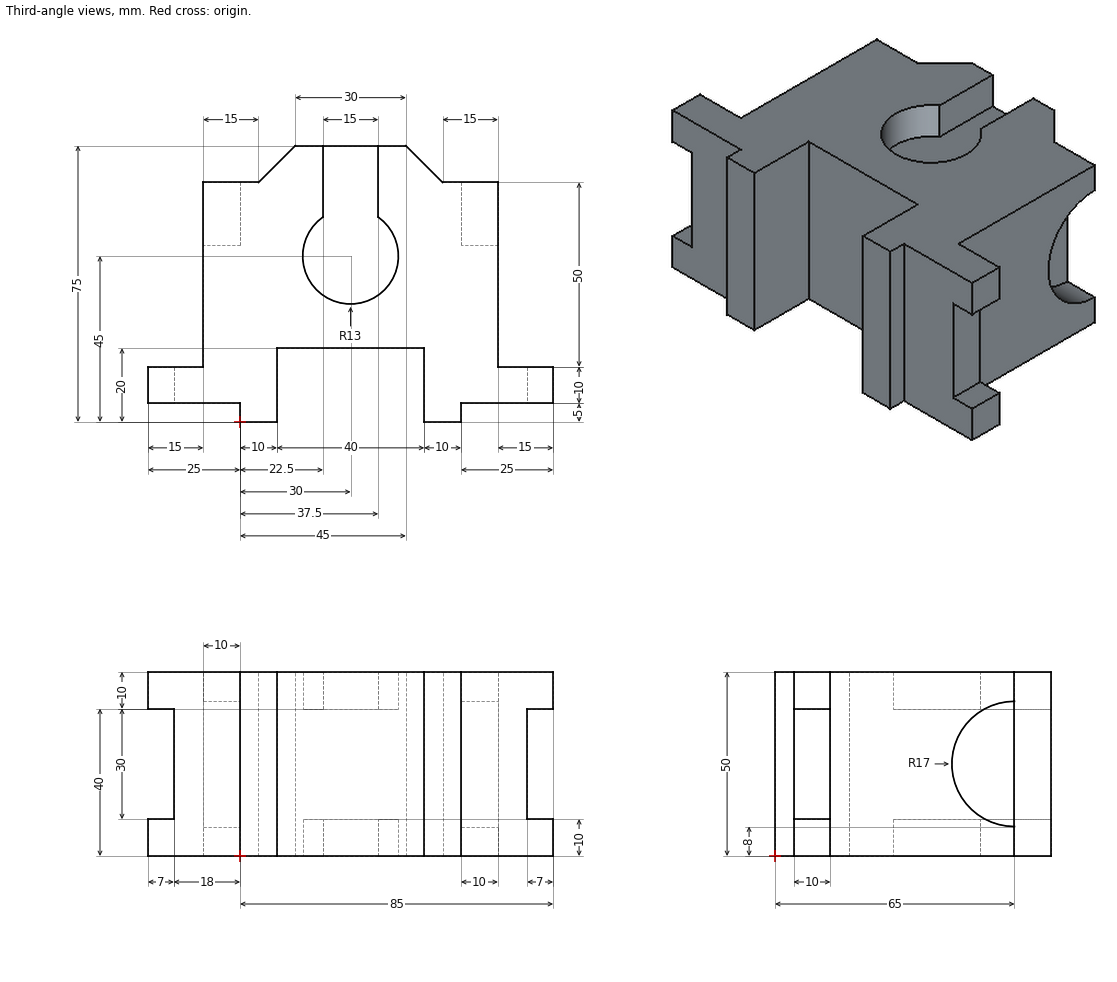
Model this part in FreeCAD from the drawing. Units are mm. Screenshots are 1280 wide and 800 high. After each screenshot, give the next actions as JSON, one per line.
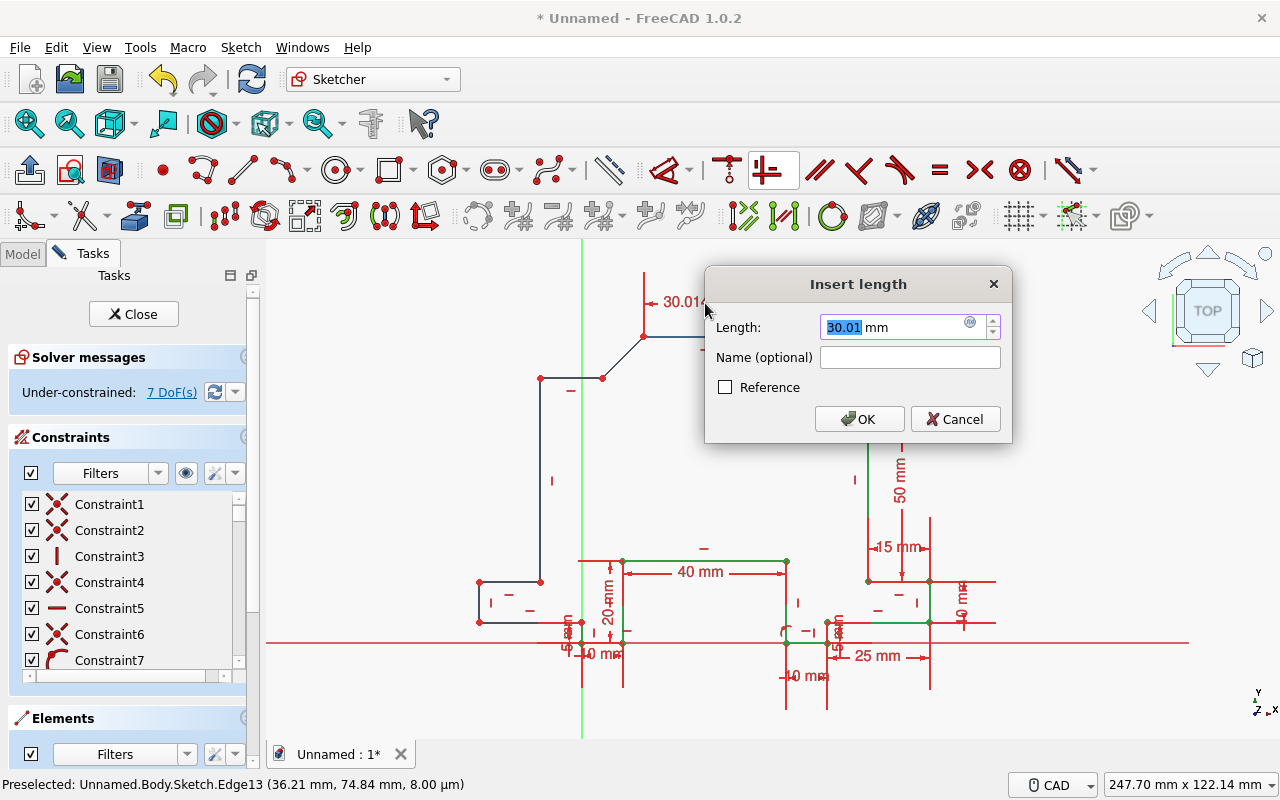
{"action": "type", "text": "30"}
{"action": "key", "text": "Return"}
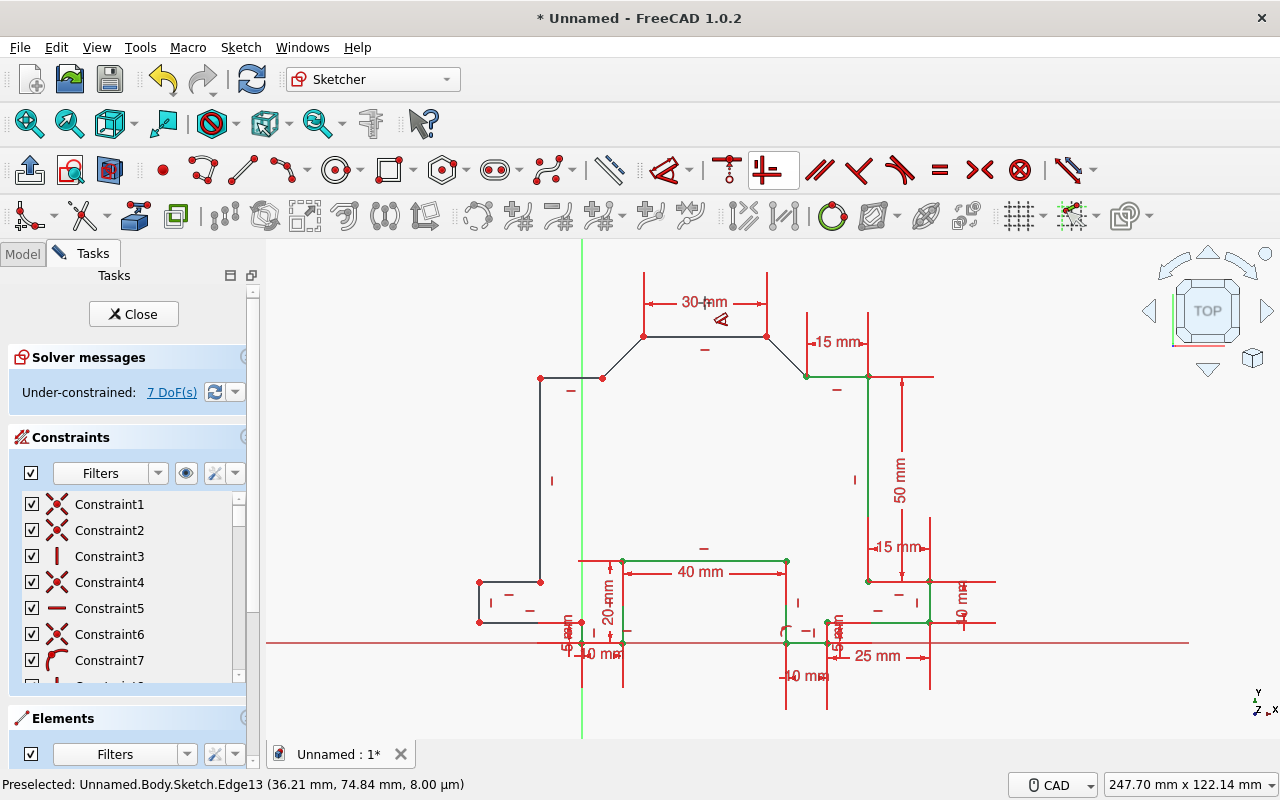
{"action": "left_click", "coordinate": [584, 378]}
{"action": "left_click", "coordinate": [557, 344]}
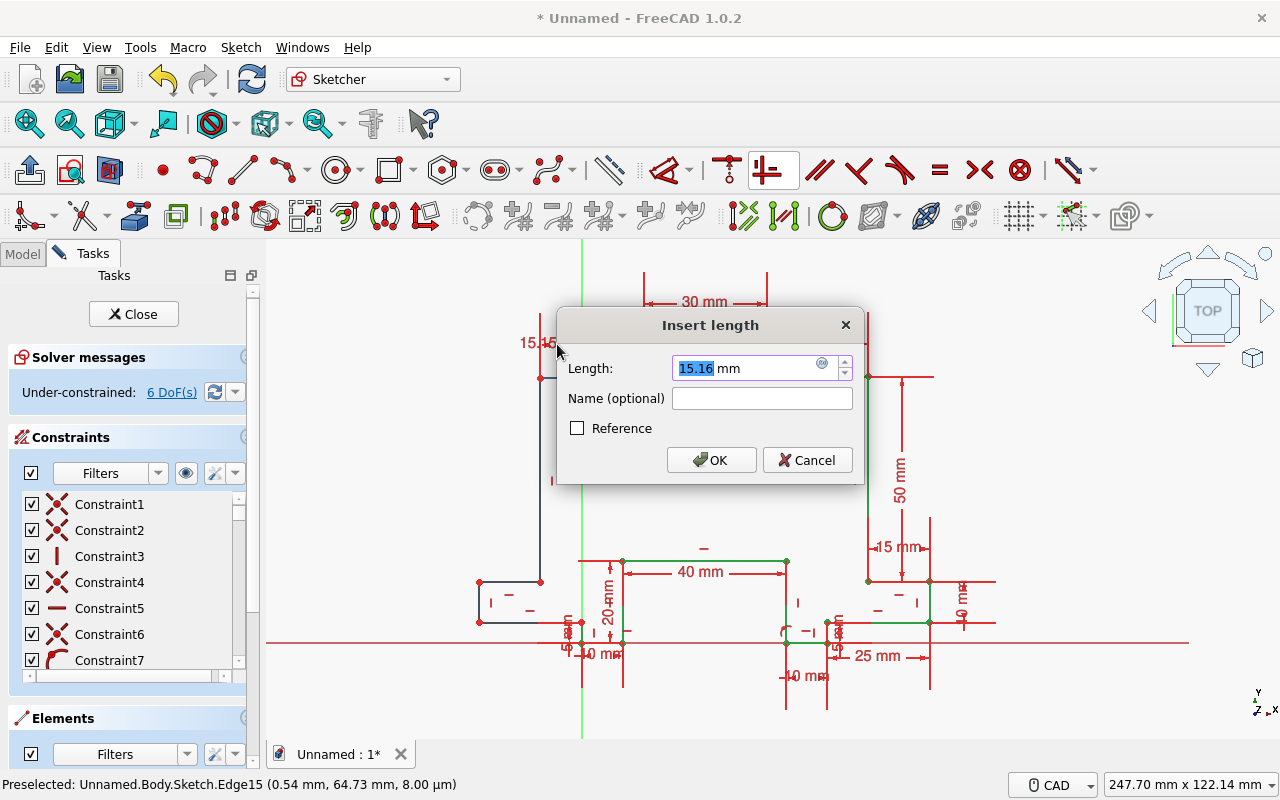
{"action": "type", "text": "15"}
{"action": "key", "text": "Return"}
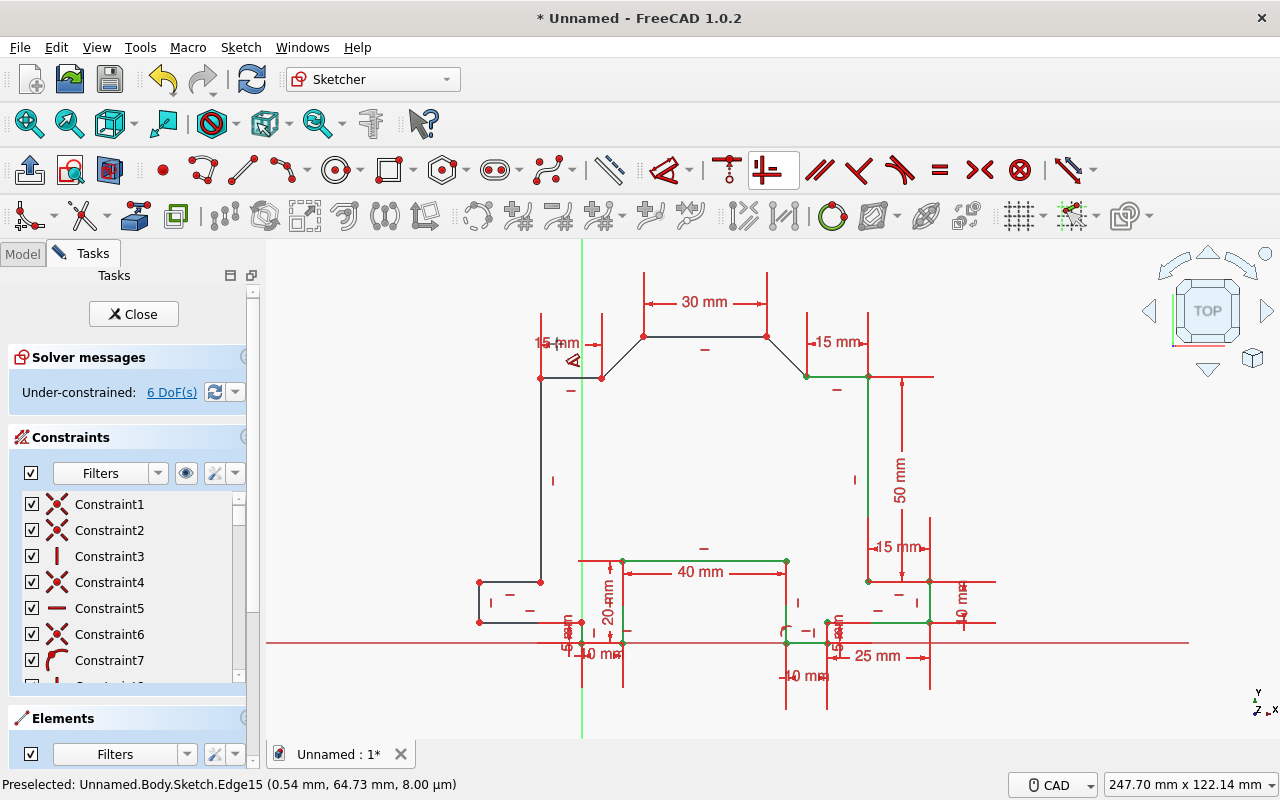
{"action": "left_click", "coordinate": [541, 439]}
{"action": "left_click", "coordinate": [507, 480]}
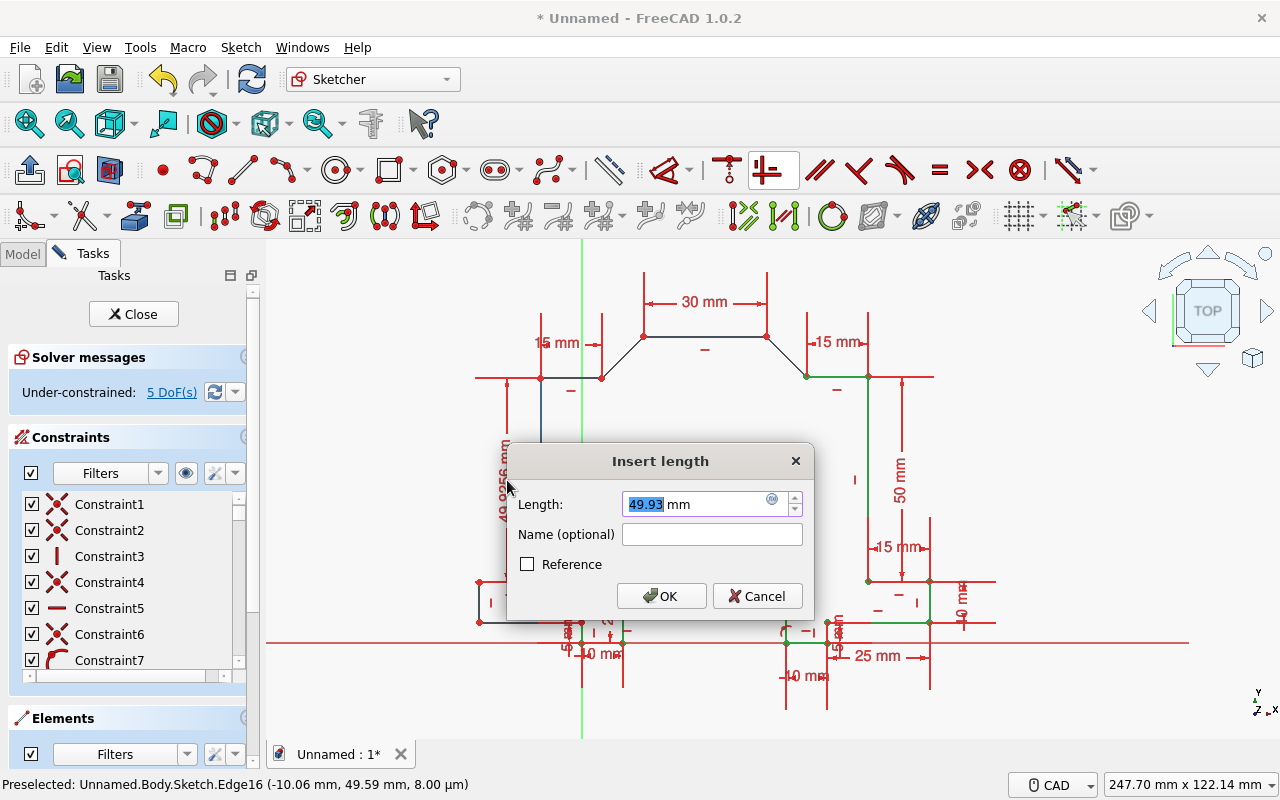
{"action": "type", "text": "50"}
{"action": "key", "text": "Return"}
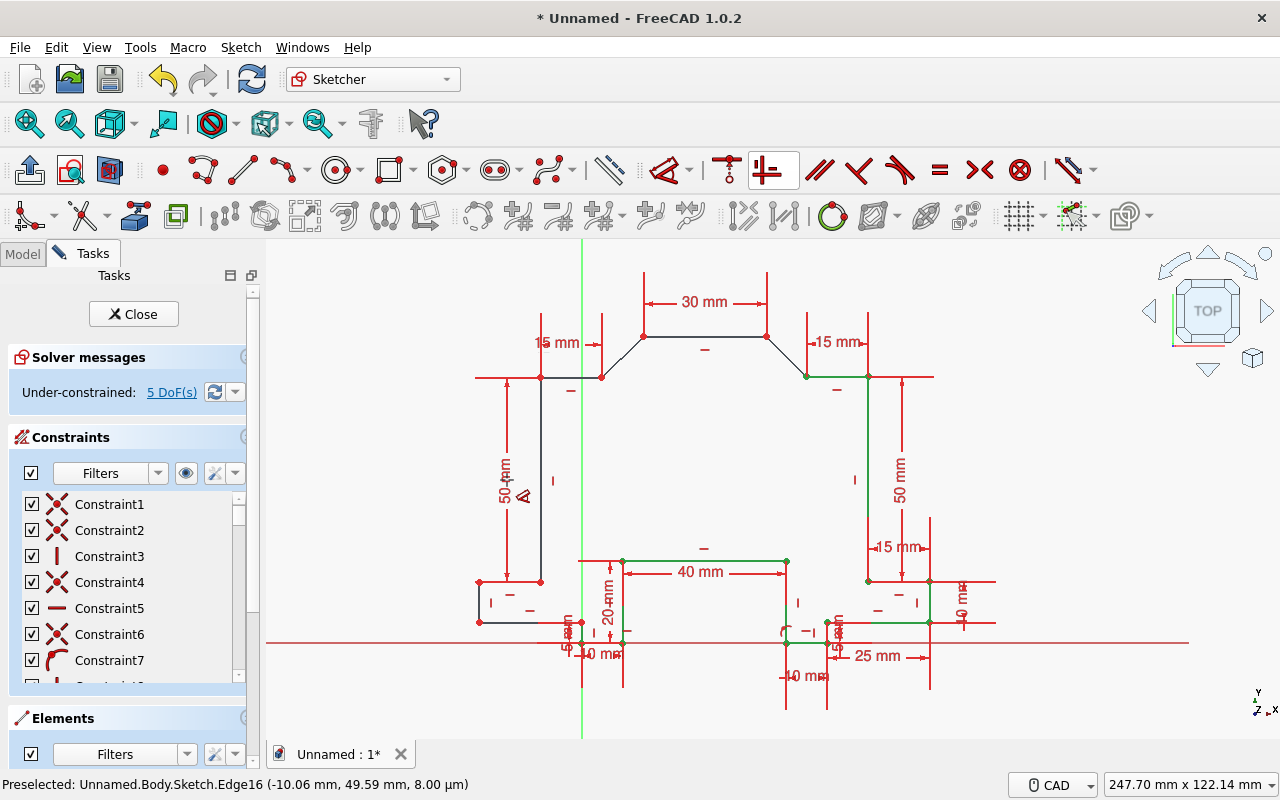
{"action": "left_click", "coordinate": [522, 582]}
{"action": "left_click", "coordinate": [510, 548]}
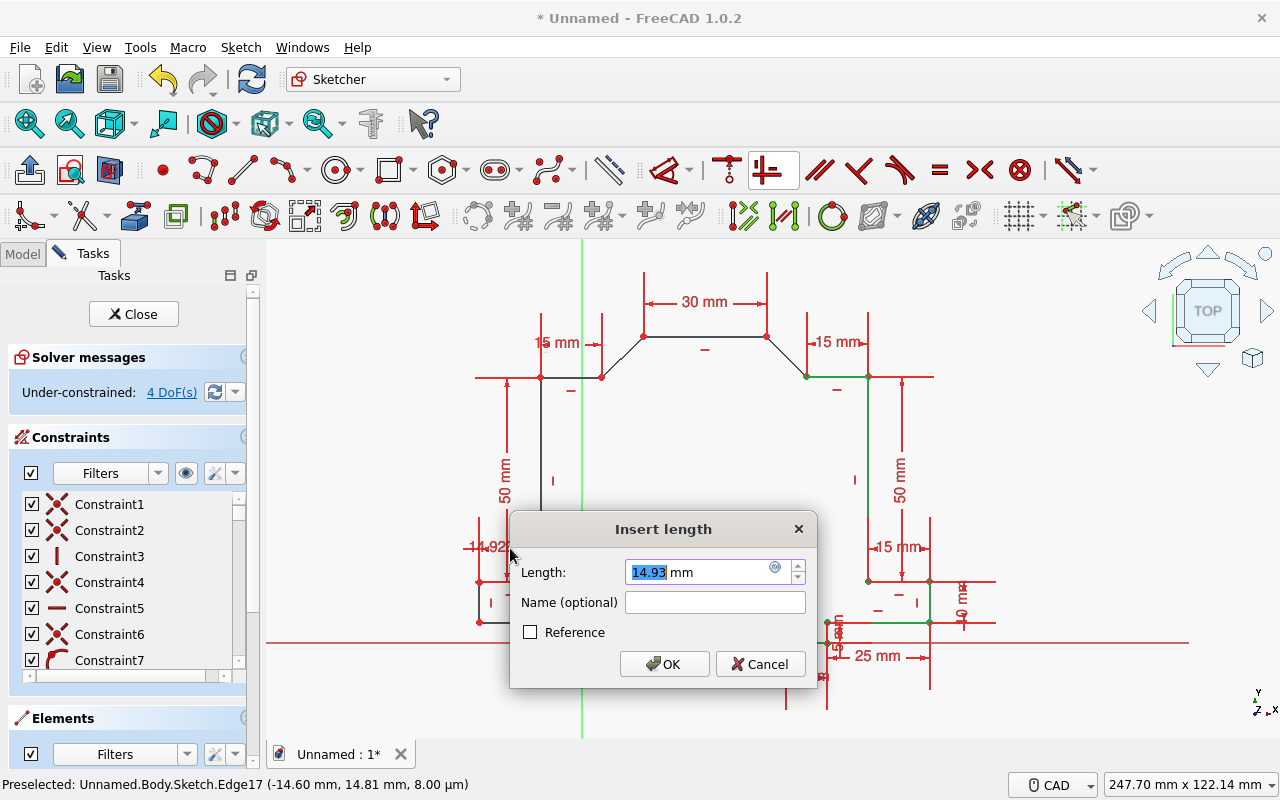
{"action": "type", "text": "15"}
{"action": "key", "text": "Return"}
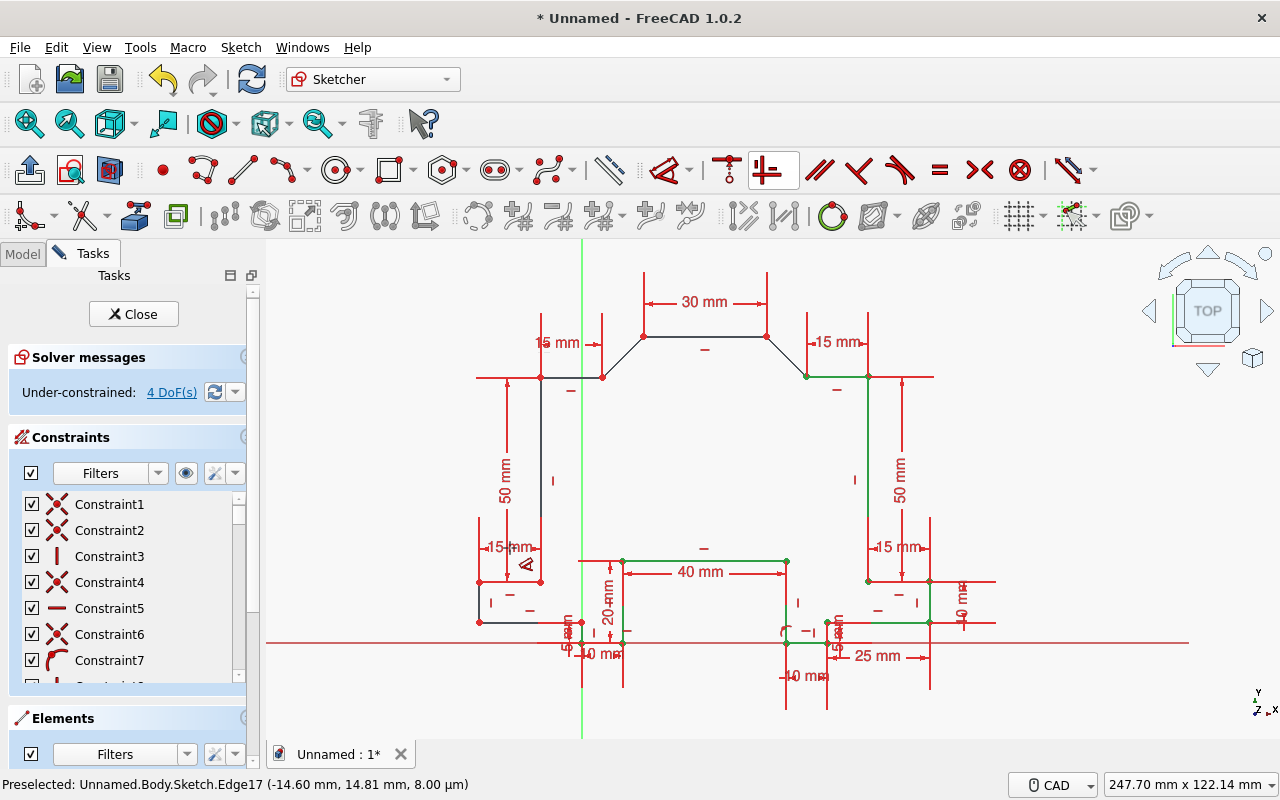
{"action": "left_click", "coordinate": [479, 594]}
{"action": "left_click", "coordinate": [445, 602]}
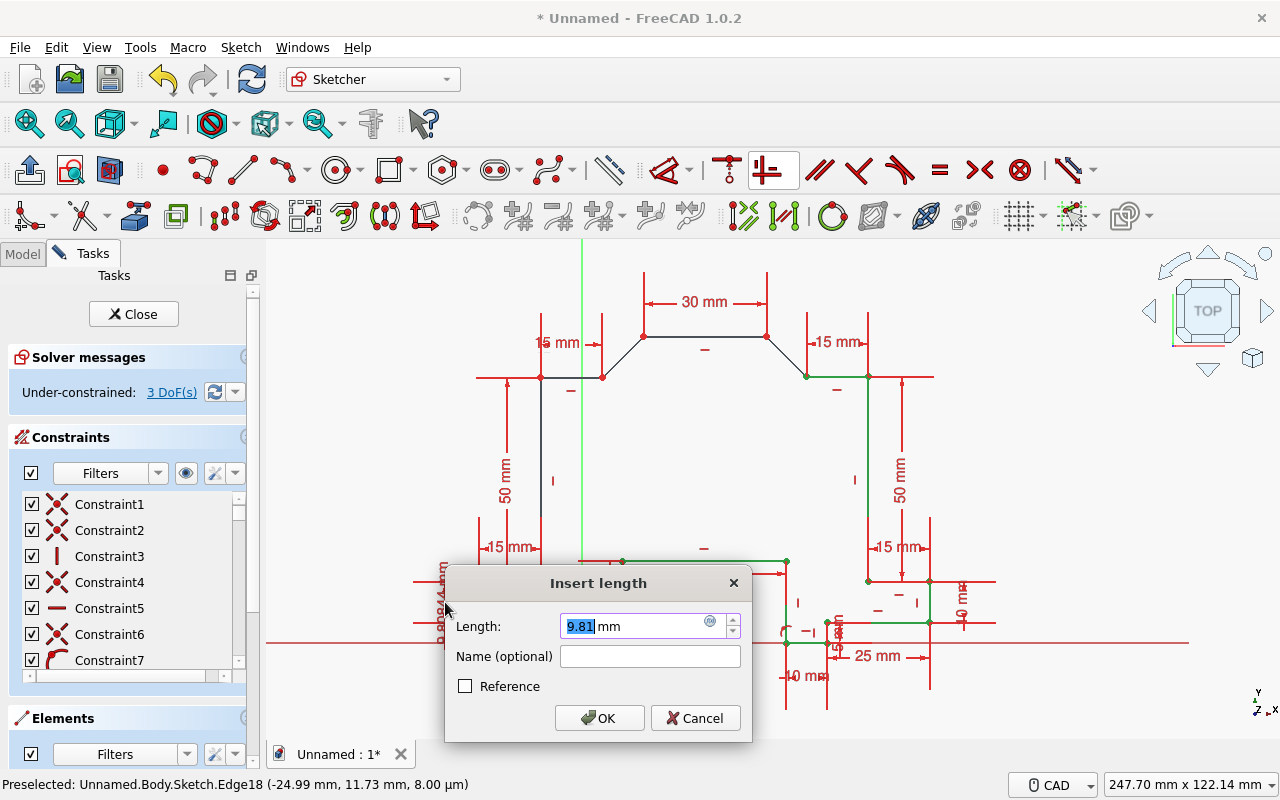
{"action": "type", "text": "10"}
{"action": "key", "text": "Return"}